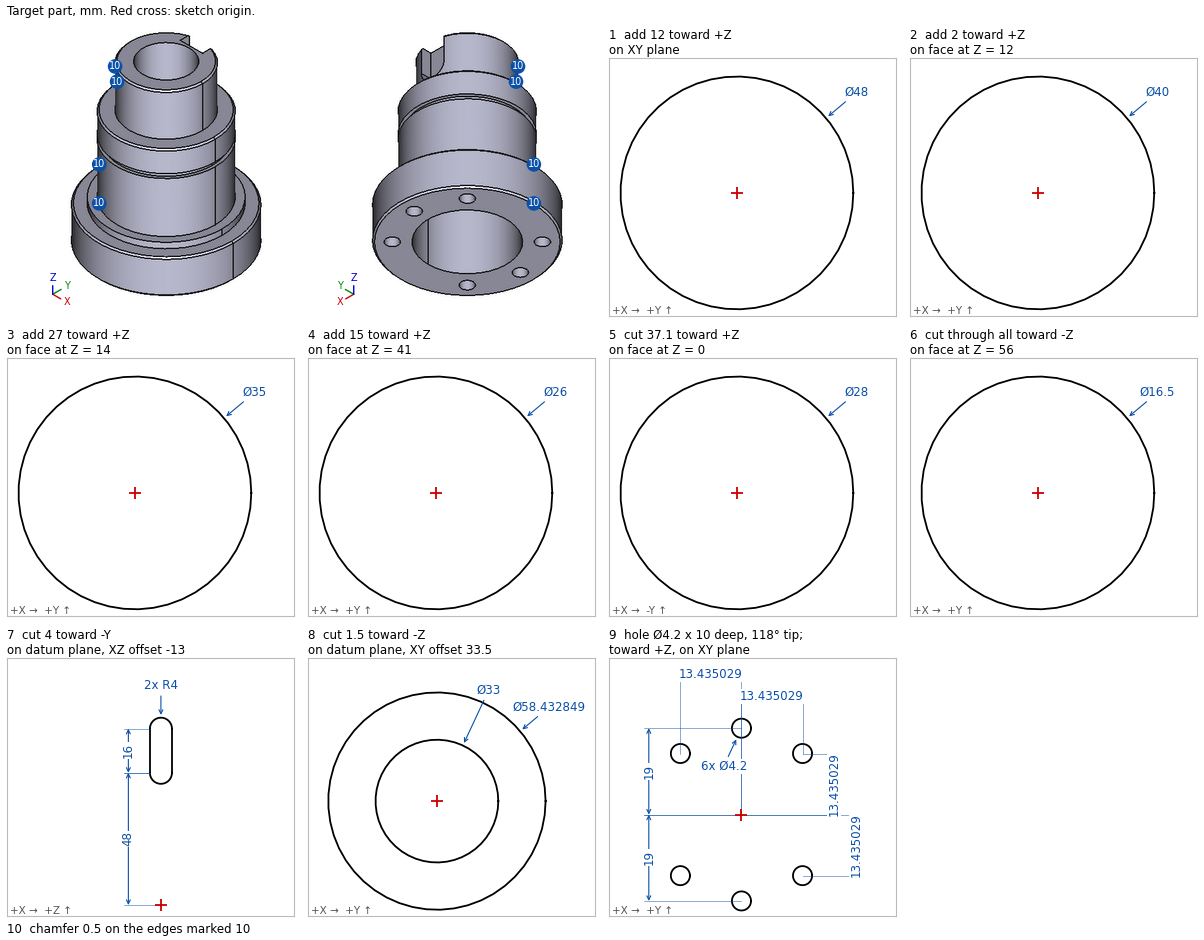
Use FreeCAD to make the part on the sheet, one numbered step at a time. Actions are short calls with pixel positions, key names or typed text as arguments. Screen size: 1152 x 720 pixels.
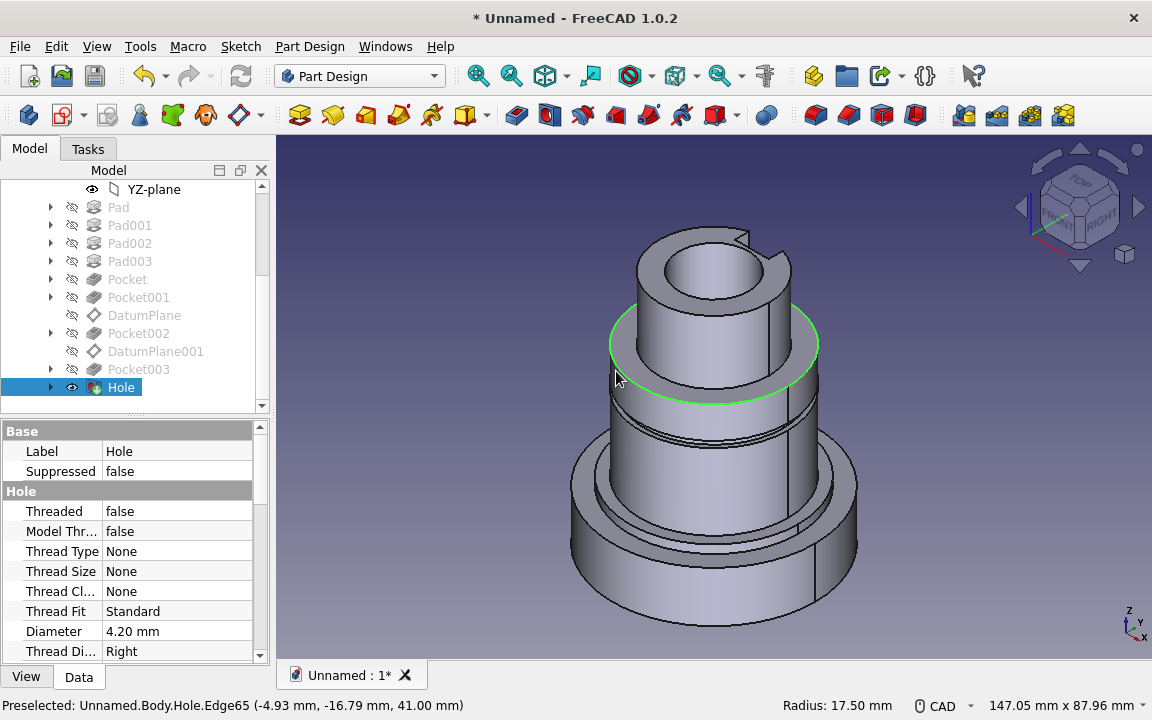
click(637, 277, ctrl)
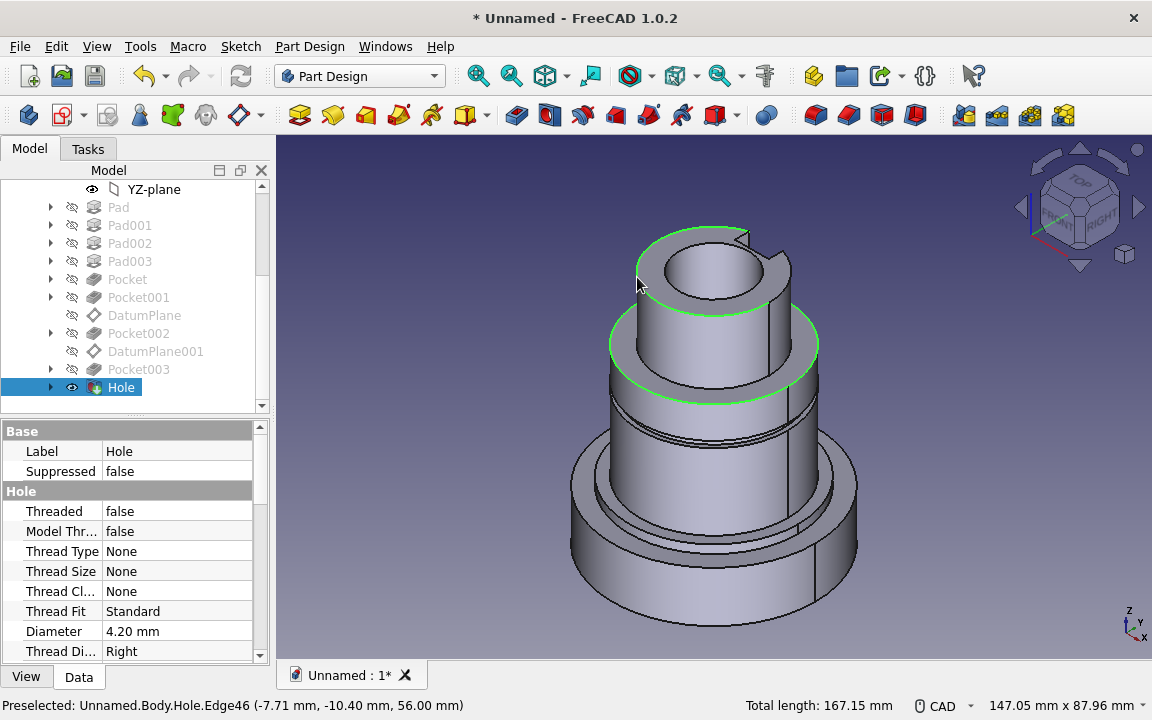
click(587, 522, ctrl)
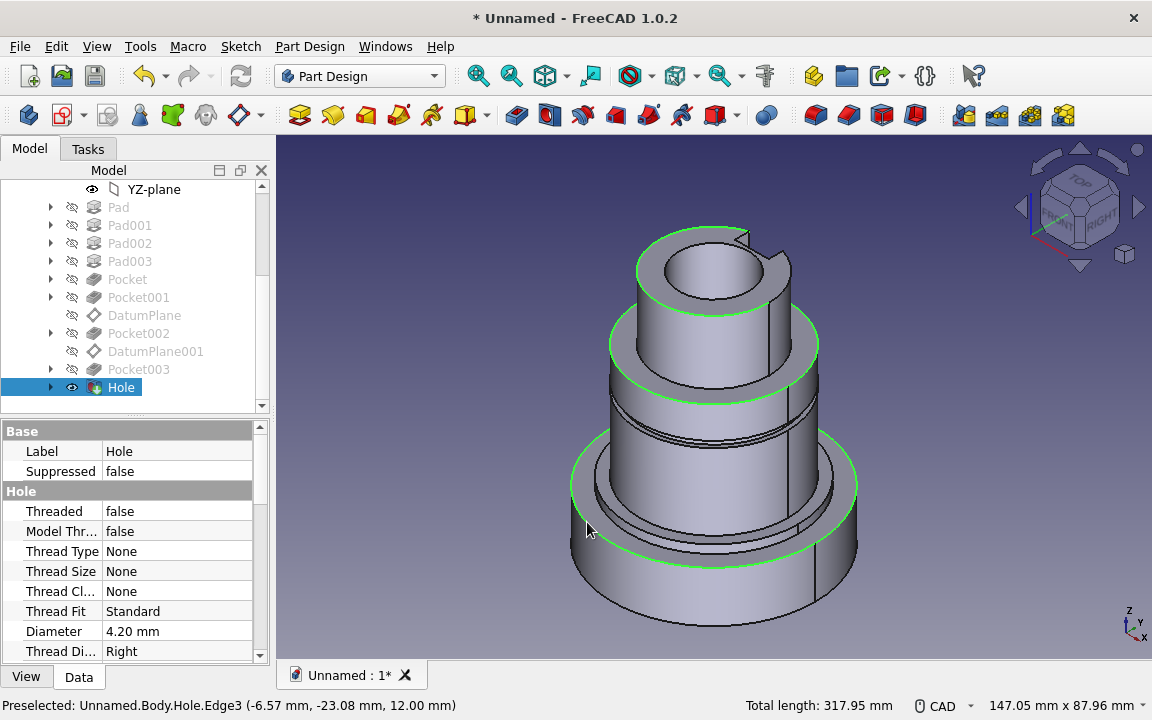
key(2)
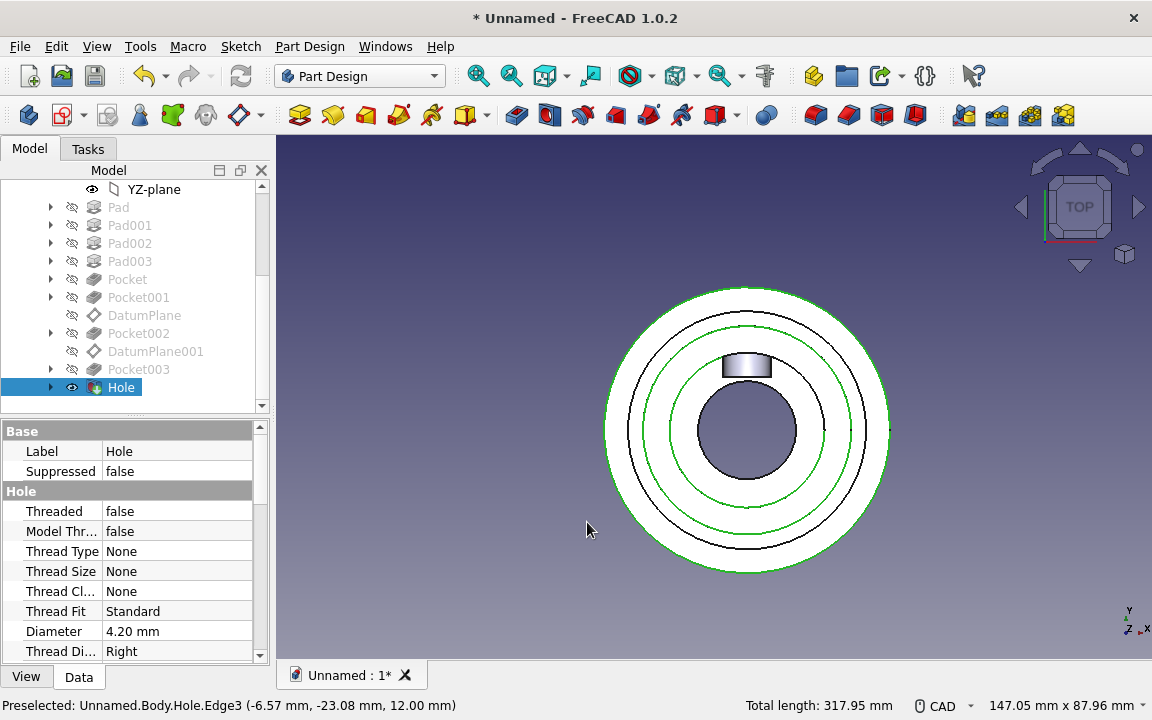
key(0)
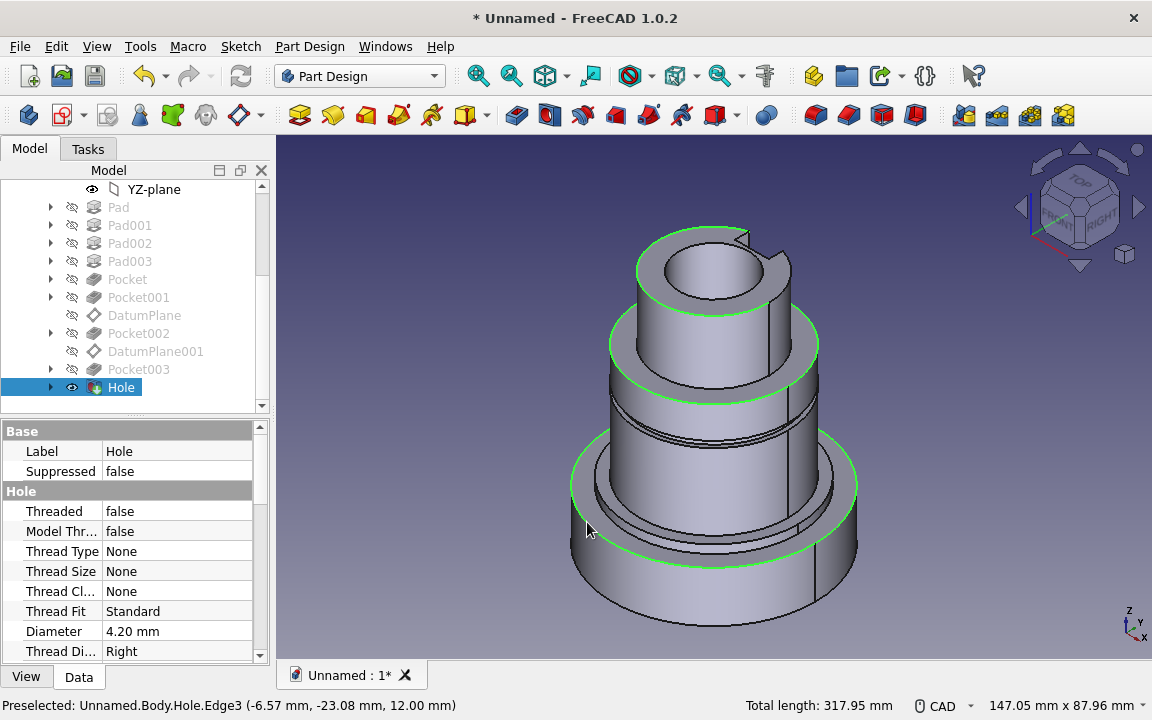
key(1)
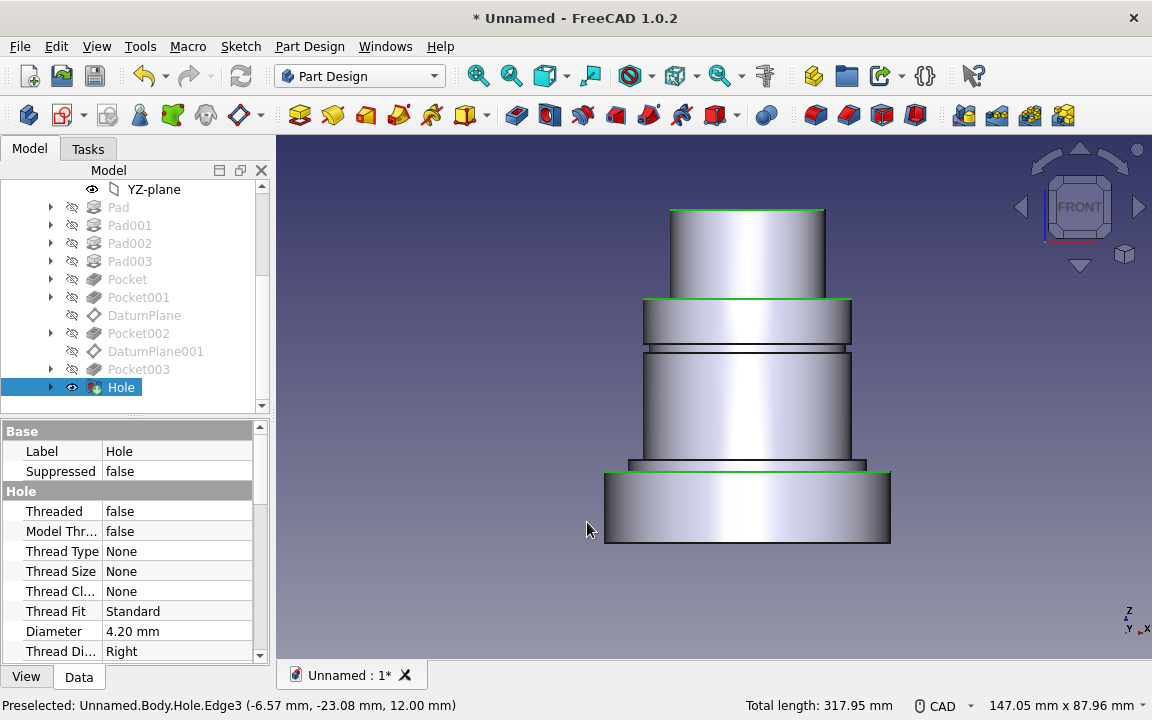
click(631, 542, ctrl)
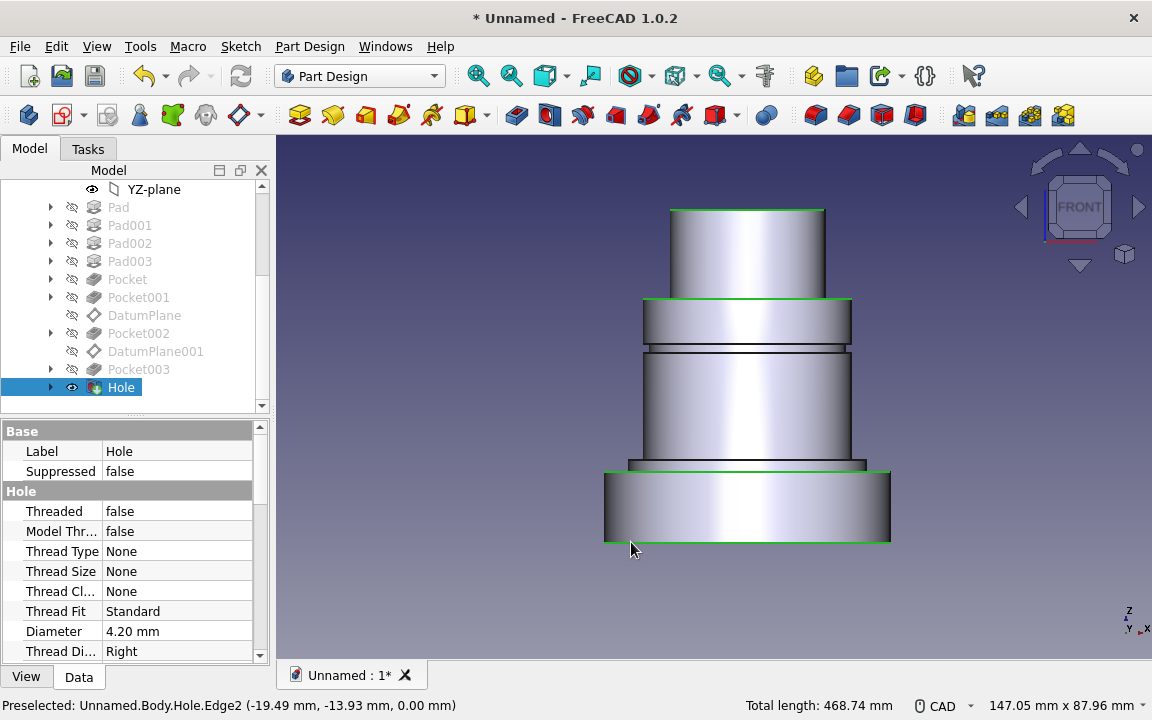
click(849, 116)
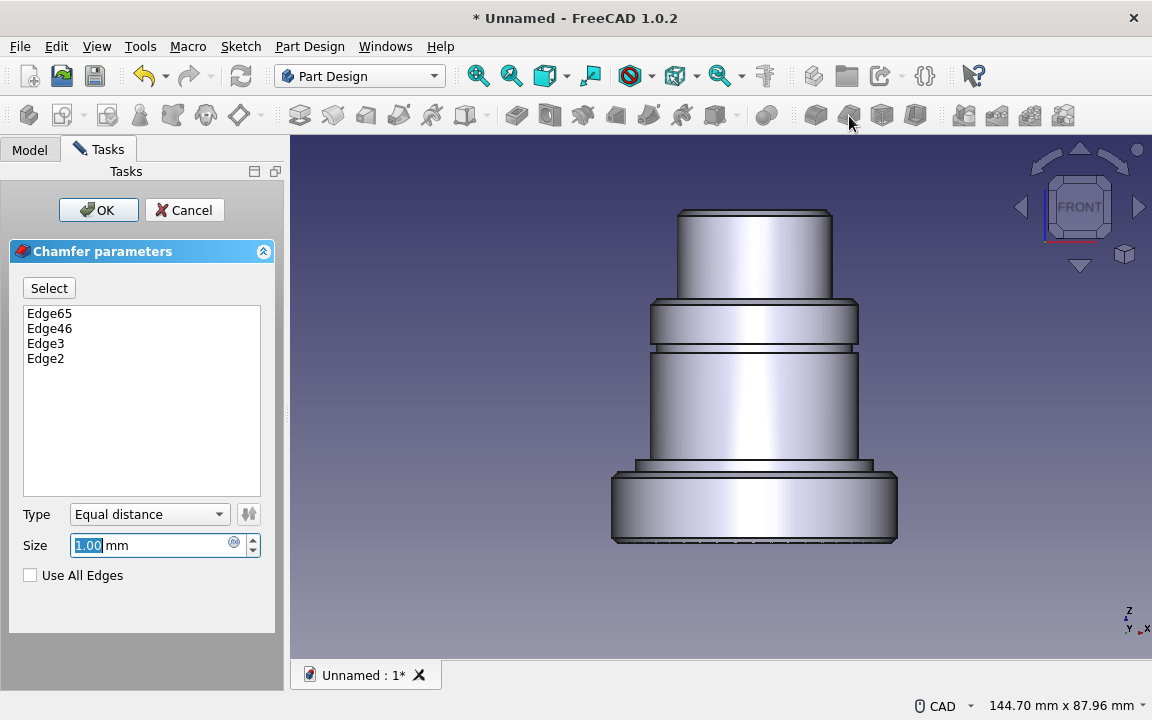
text(0.5)
key(Tab)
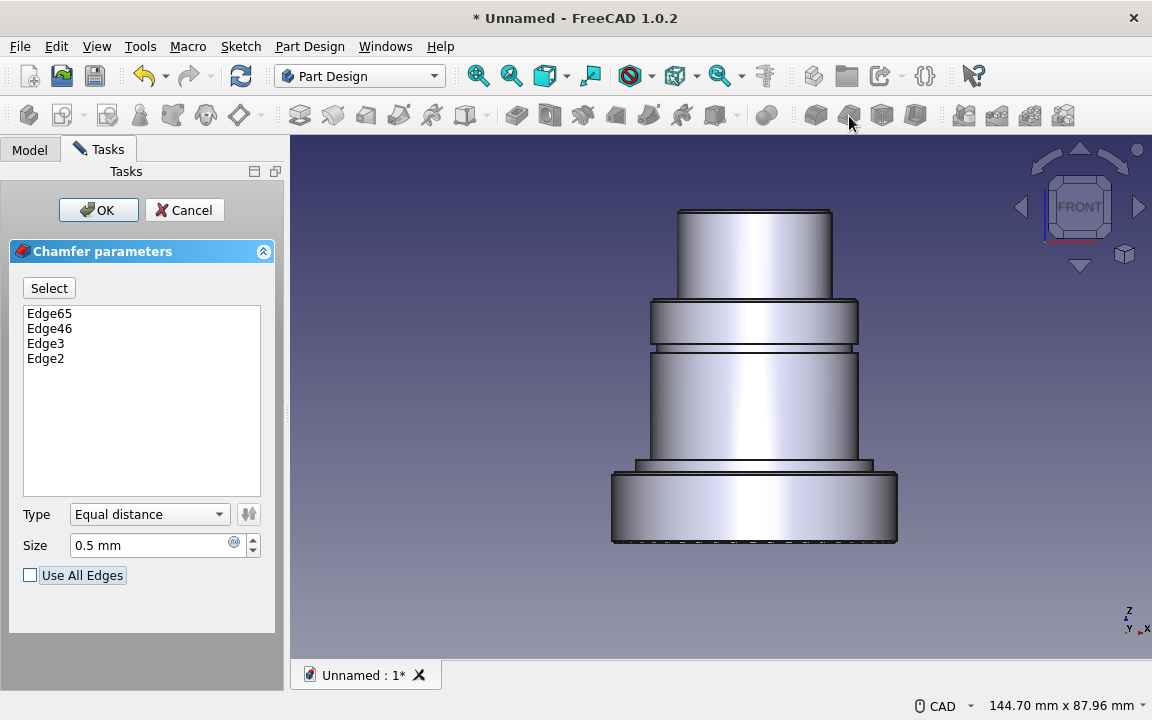
click(99, 210)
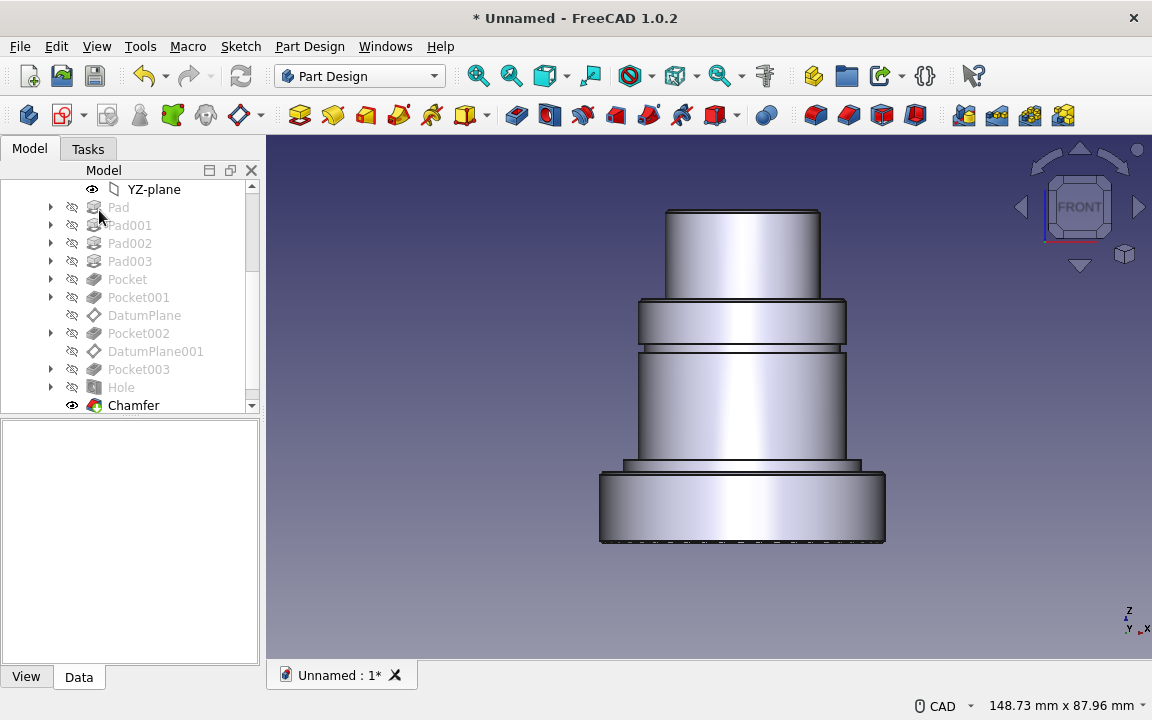
key(0)